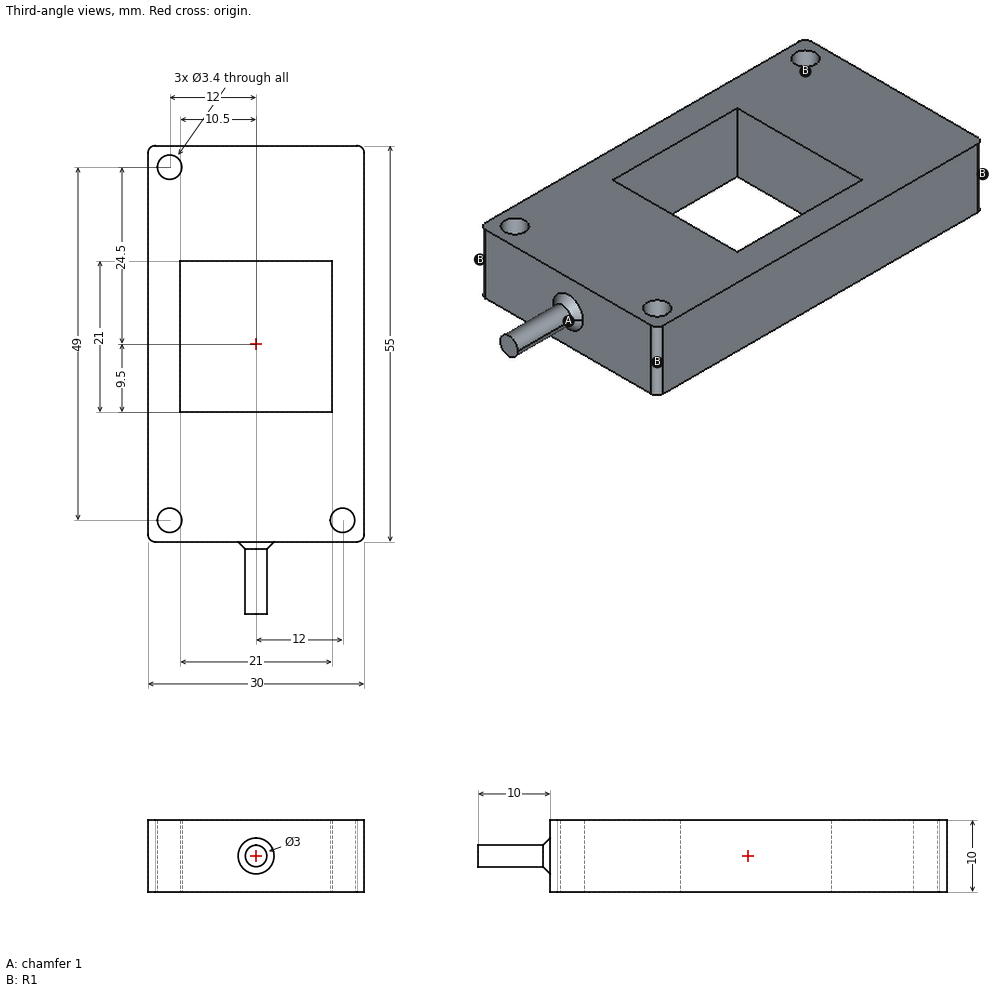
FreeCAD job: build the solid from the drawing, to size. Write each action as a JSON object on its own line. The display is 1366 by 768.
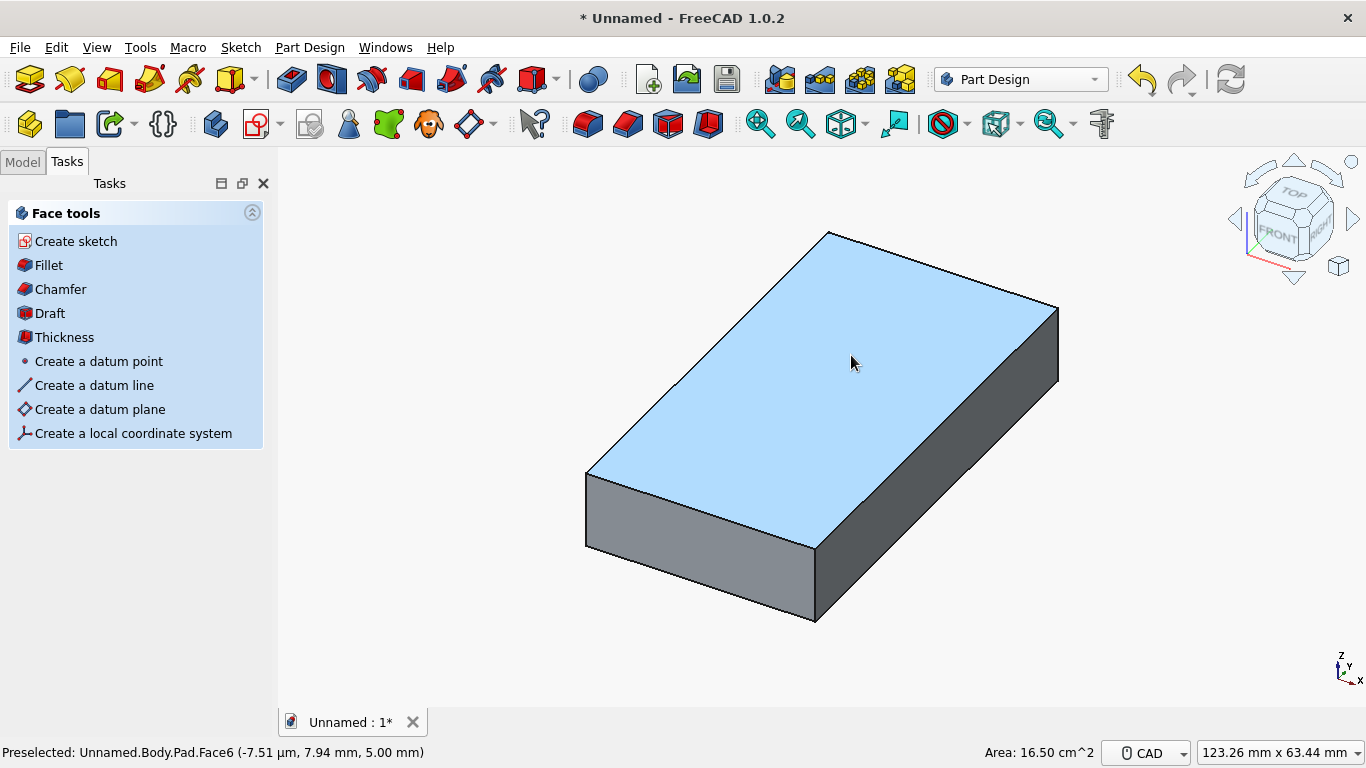
{"action": "left_click", "coordinate": [256, 124]}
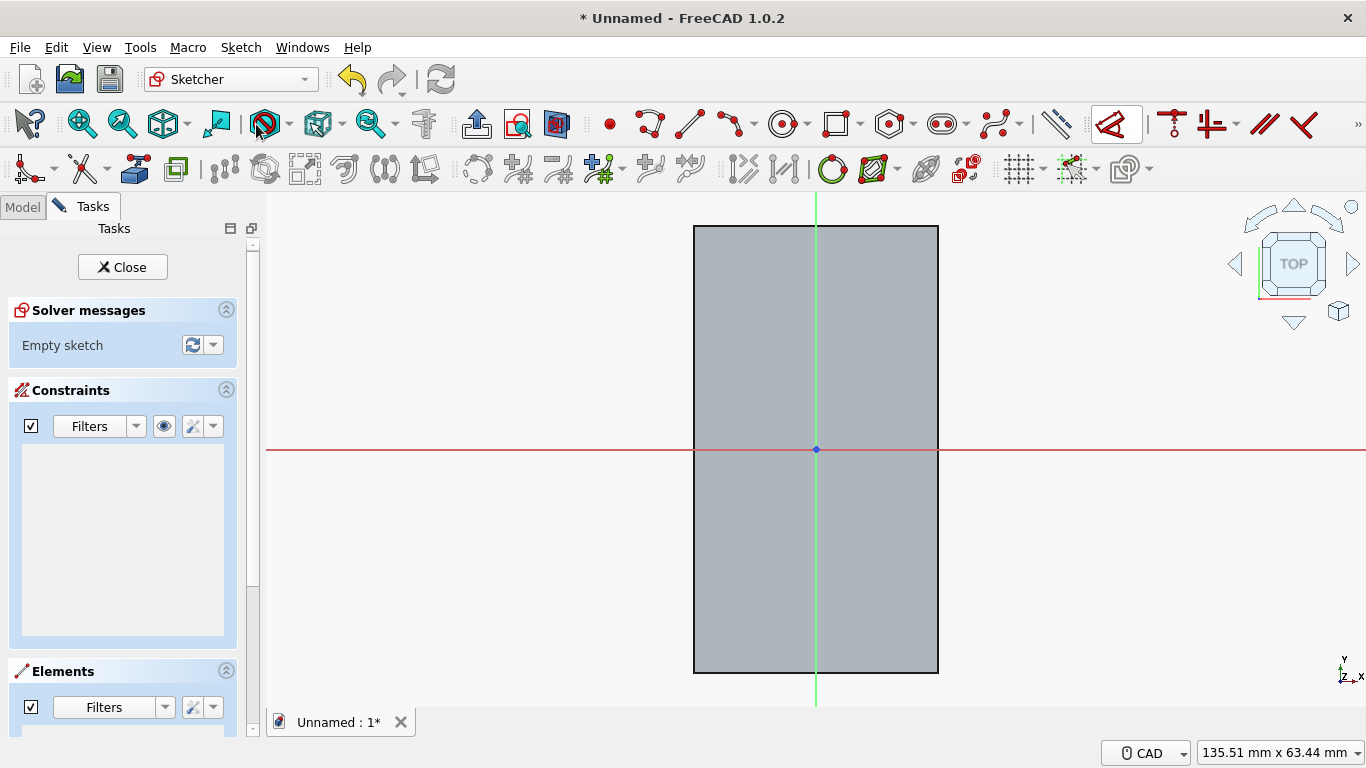
{"action": "scroll", "coordinate": [899, 432], "scroll_direction": "up", "scroll_amount": 3}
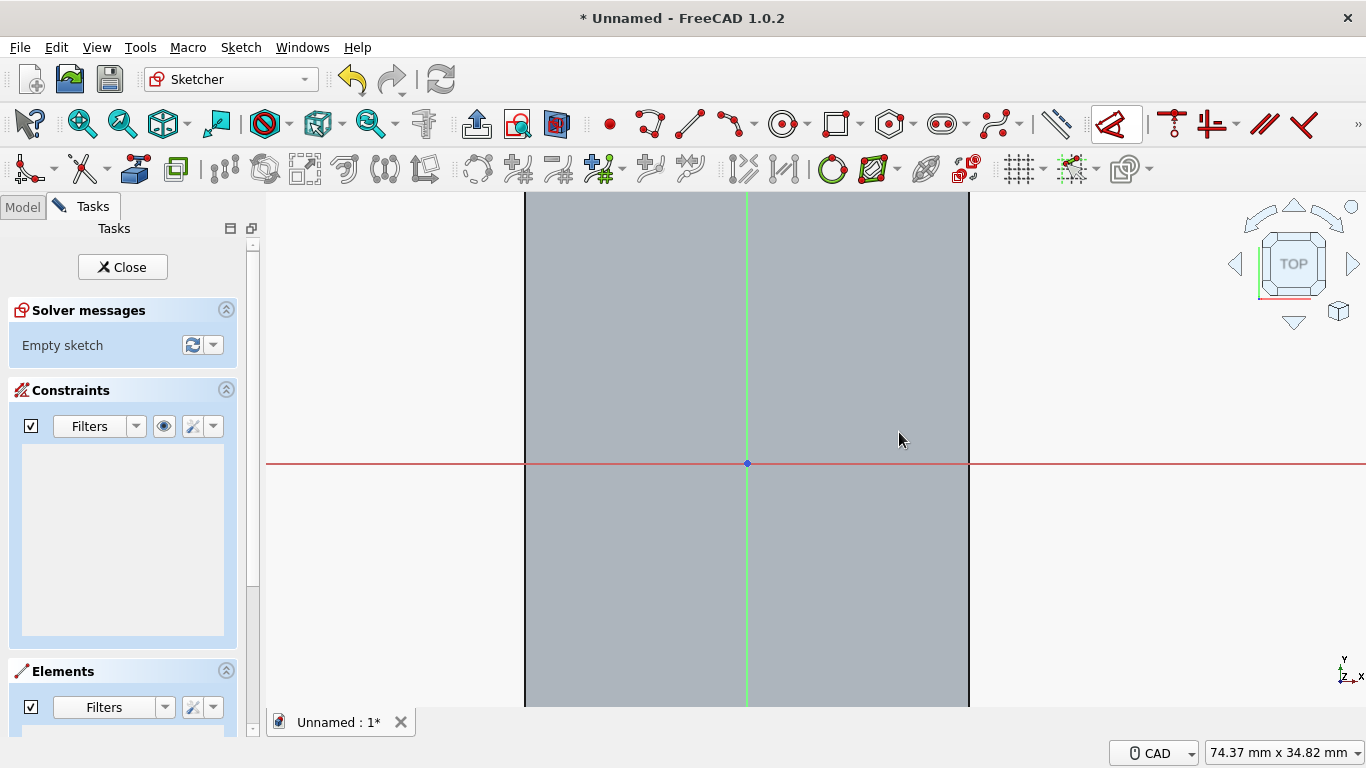
{"action": "key", "text": "g r"}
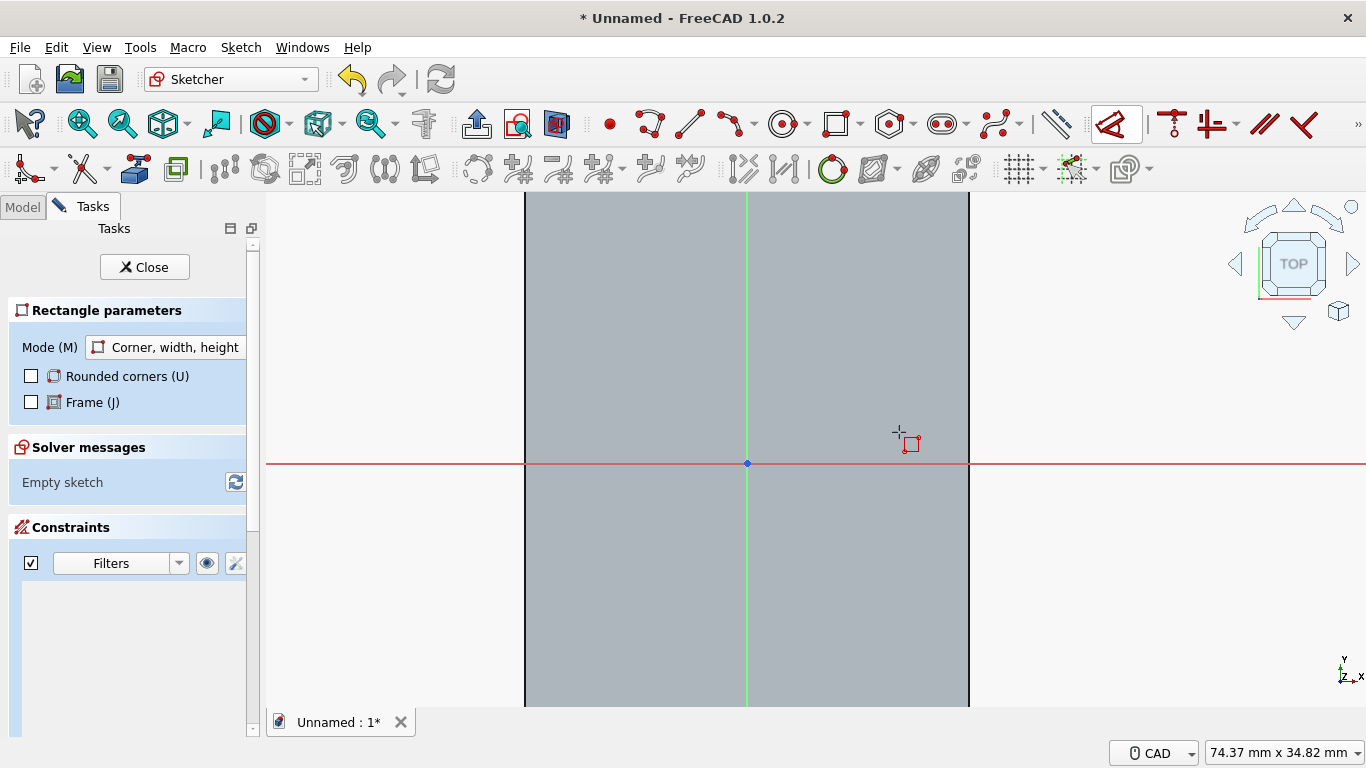
{"action": "left_click", "coordinate": [592, 293]}
{"action": "left_click", "coordinate": [903, 604]}
{"action": "key", "text": "Escape"}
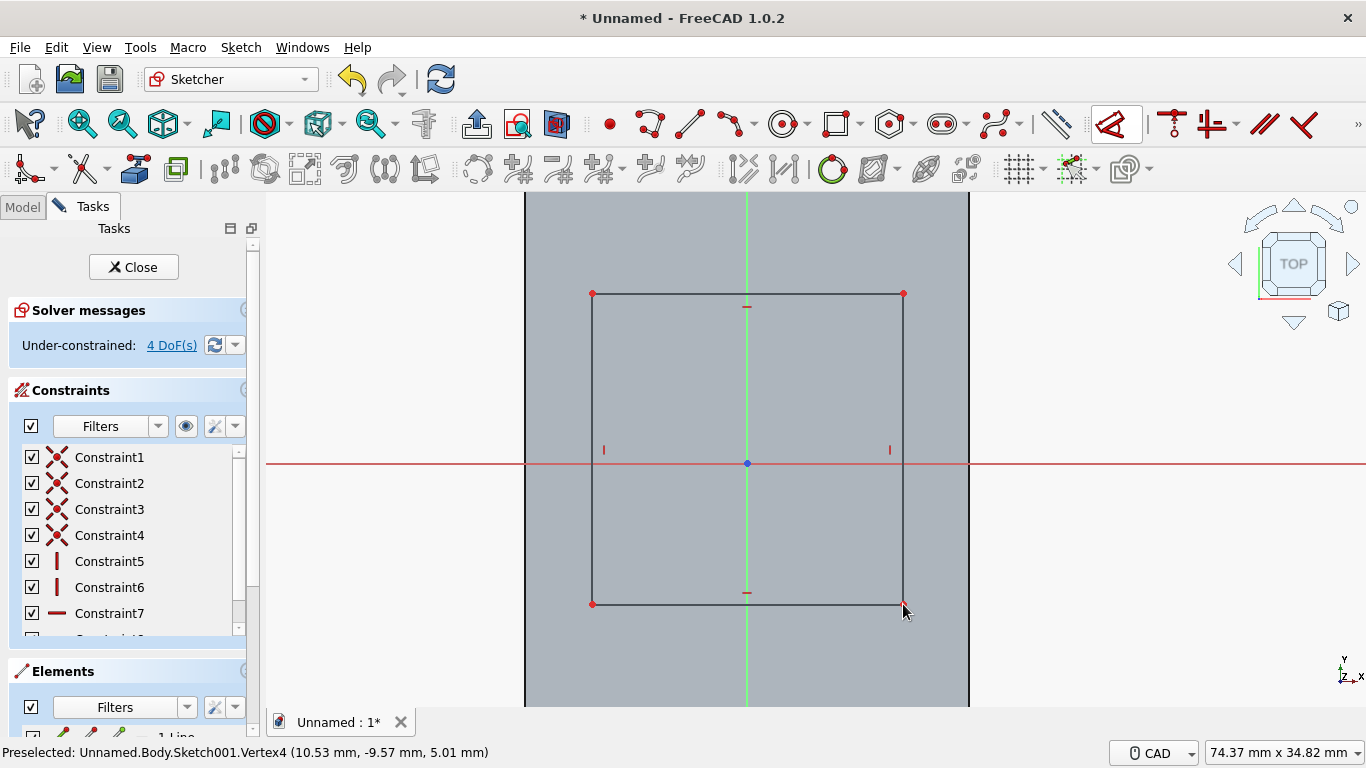
{"action": "key", "text": "d"}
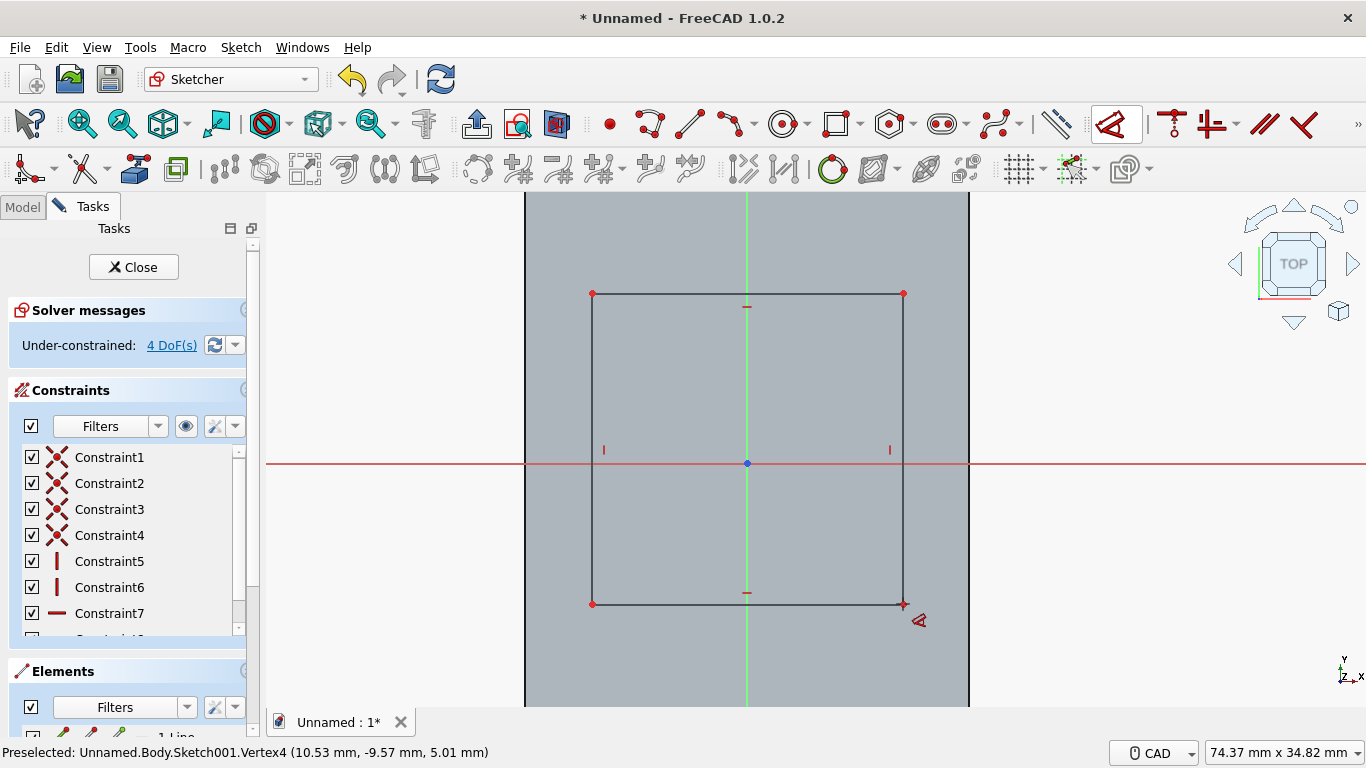
{"action": "left_click", "coordinate": [592, 387]}
{"action": "left_click", "coordinate": [558, 450]}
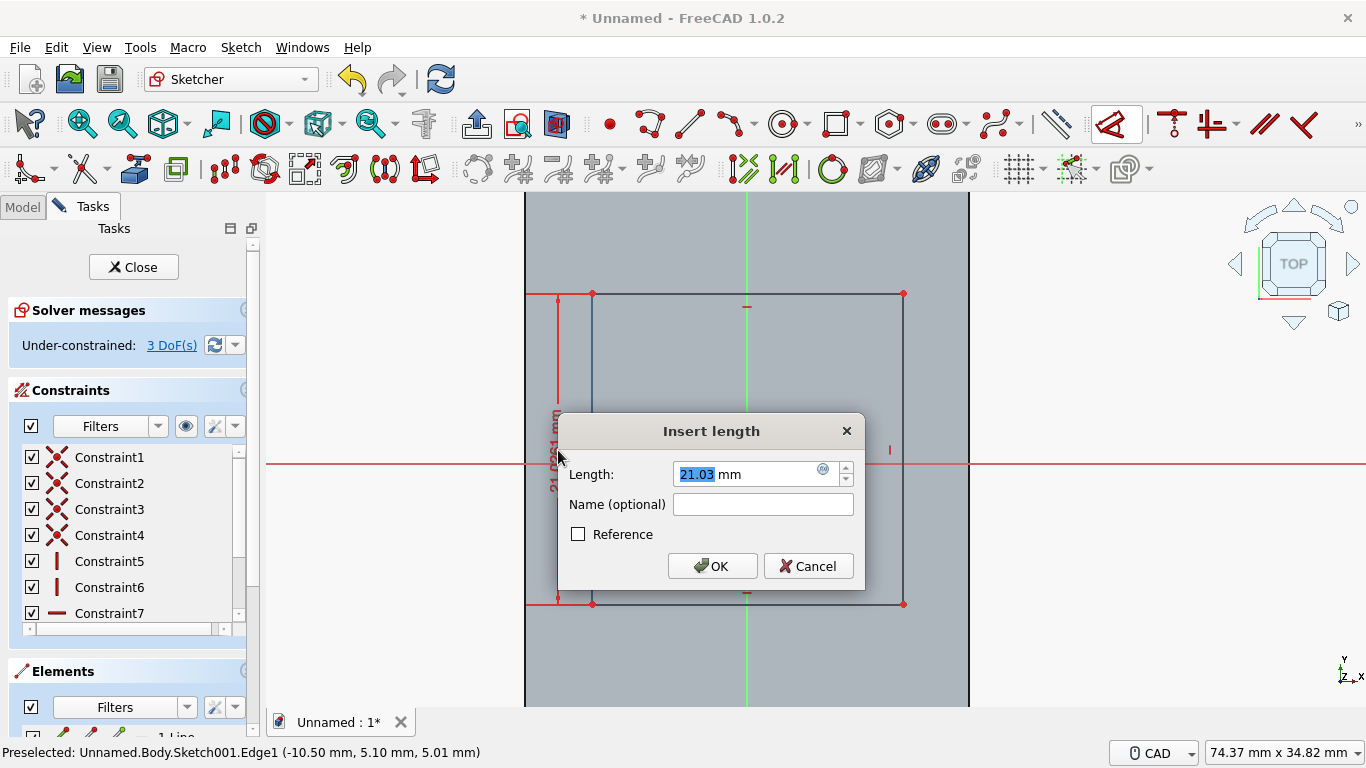
{"action": "type", "text": "21"}
{"action": "key", "text": "Return"}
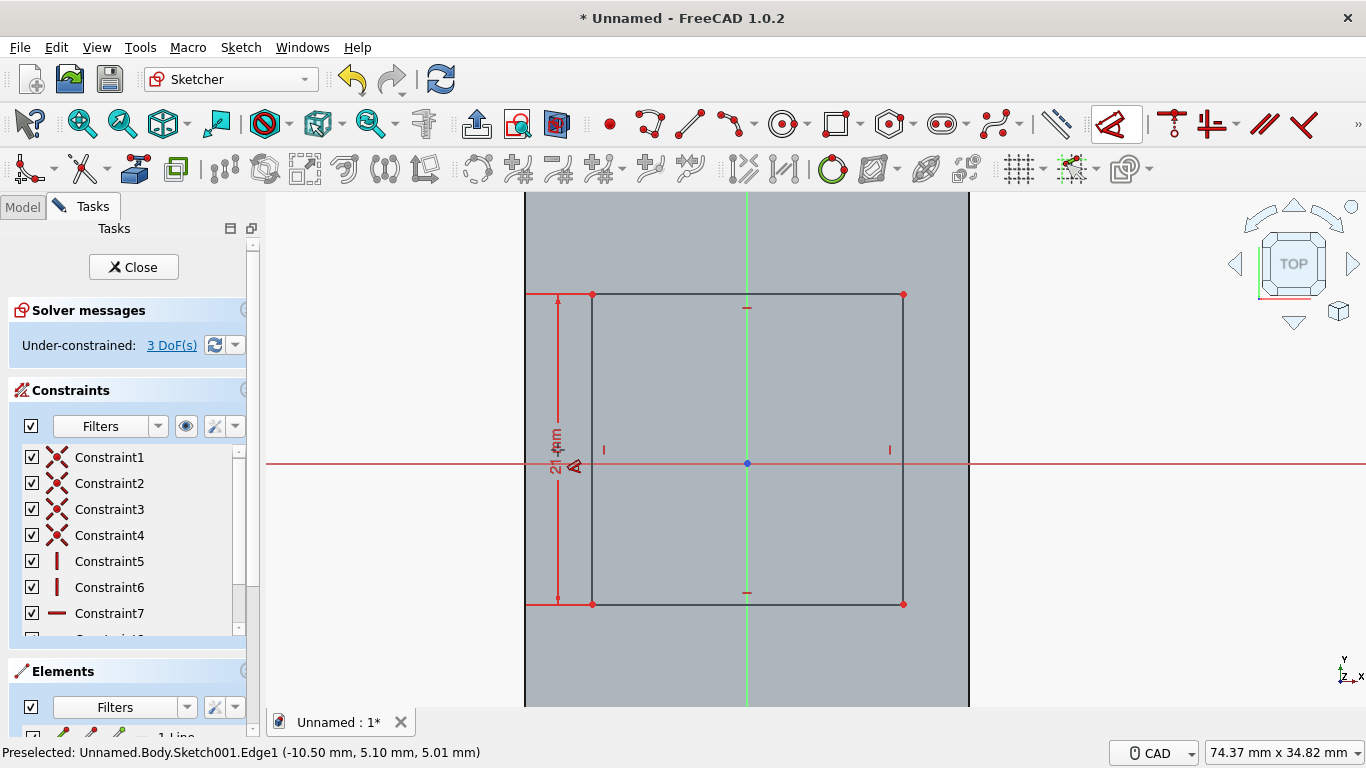
{"action": "left_click", "coordinate": [685, 605]}
{"action": "left_click", "coordinate": [676, 639]}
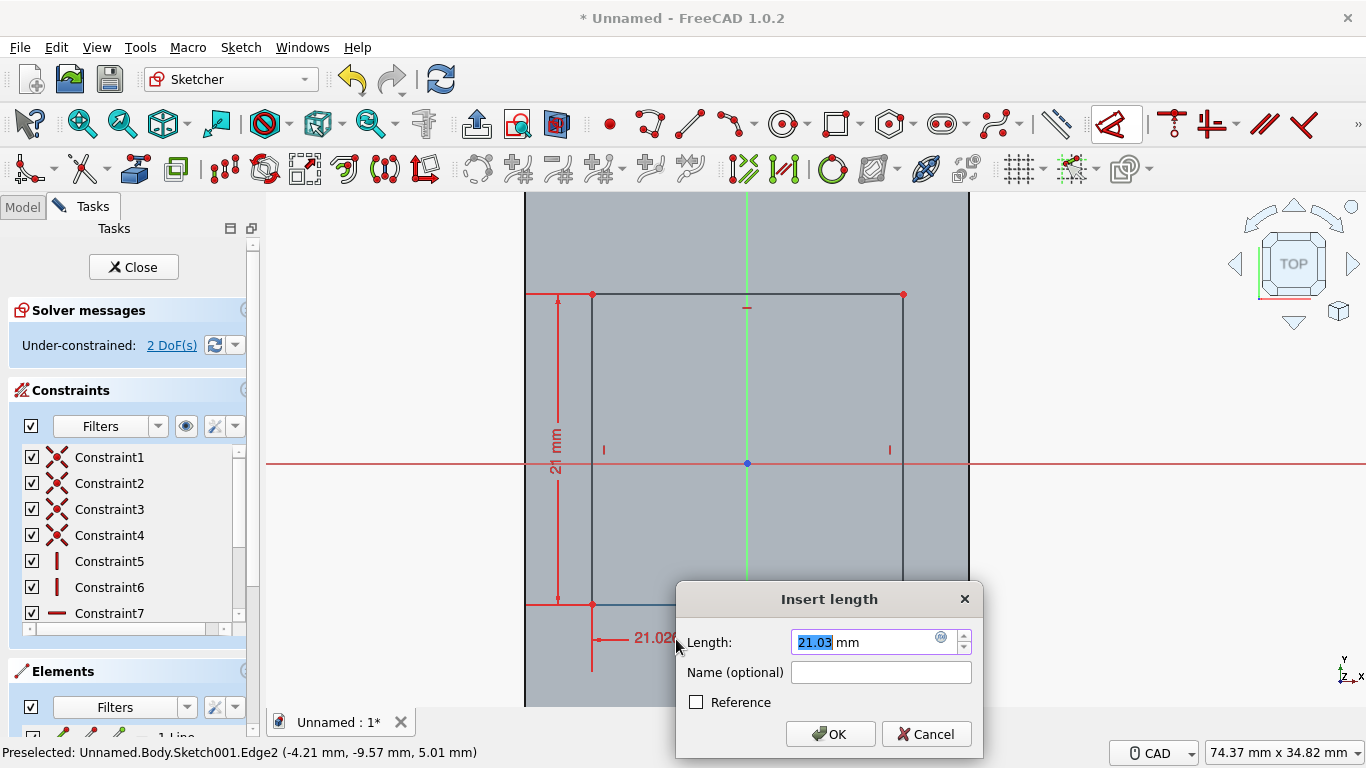
{"action": "type", "text": "21"}
{"action": "key", "text": "Return"}